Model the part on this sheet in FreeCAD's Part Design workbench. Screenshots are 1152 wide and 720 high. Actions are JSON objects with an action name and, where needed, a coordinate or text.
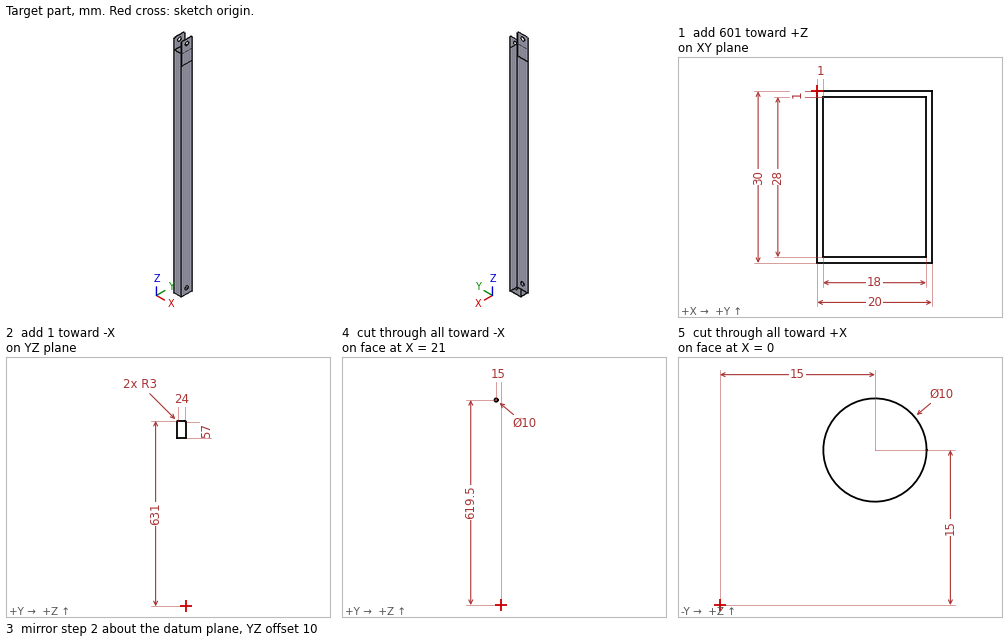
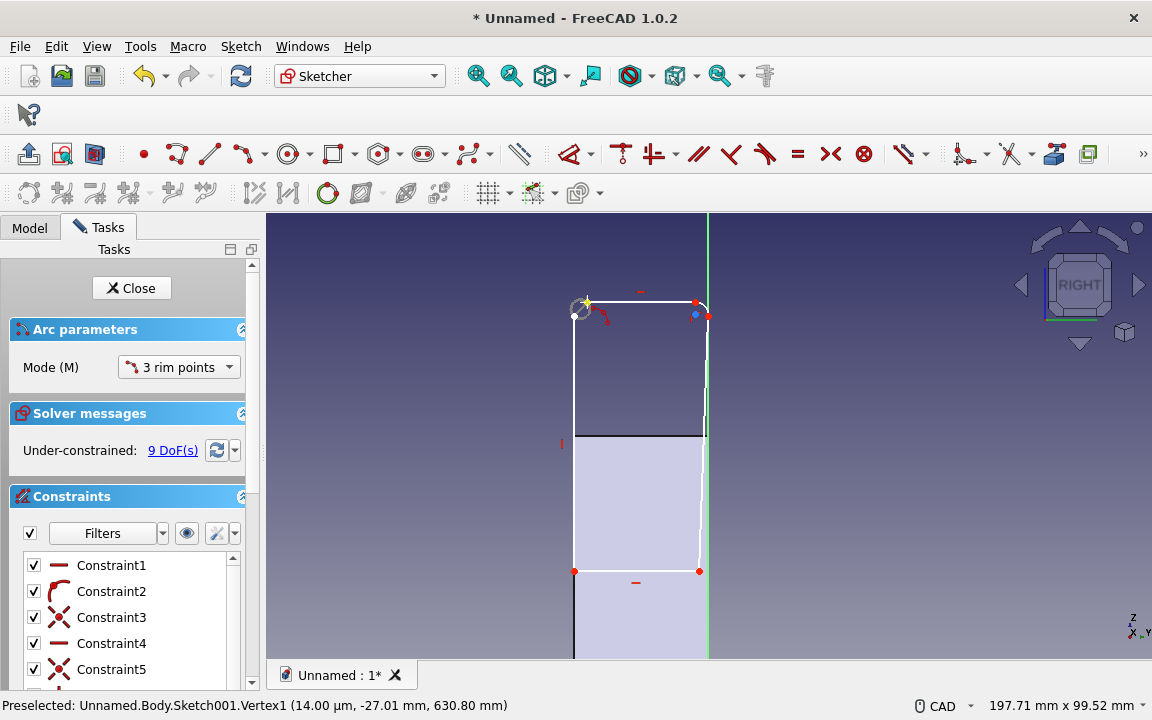
{"action": "scroll", "coordinate": [578, 305], "scroll_direction": "up", "scroll_amount": 7}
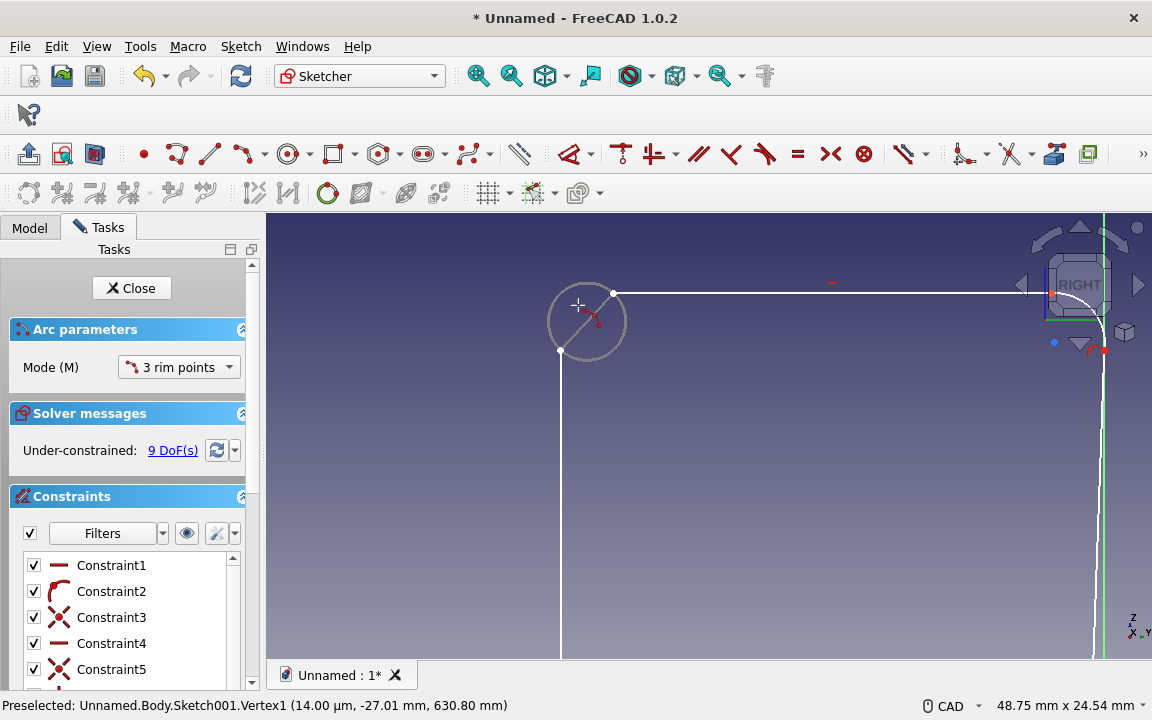
{"action": "left_click", "coordinate": [575, 306]}
{"action": "key", "text": "Escape"}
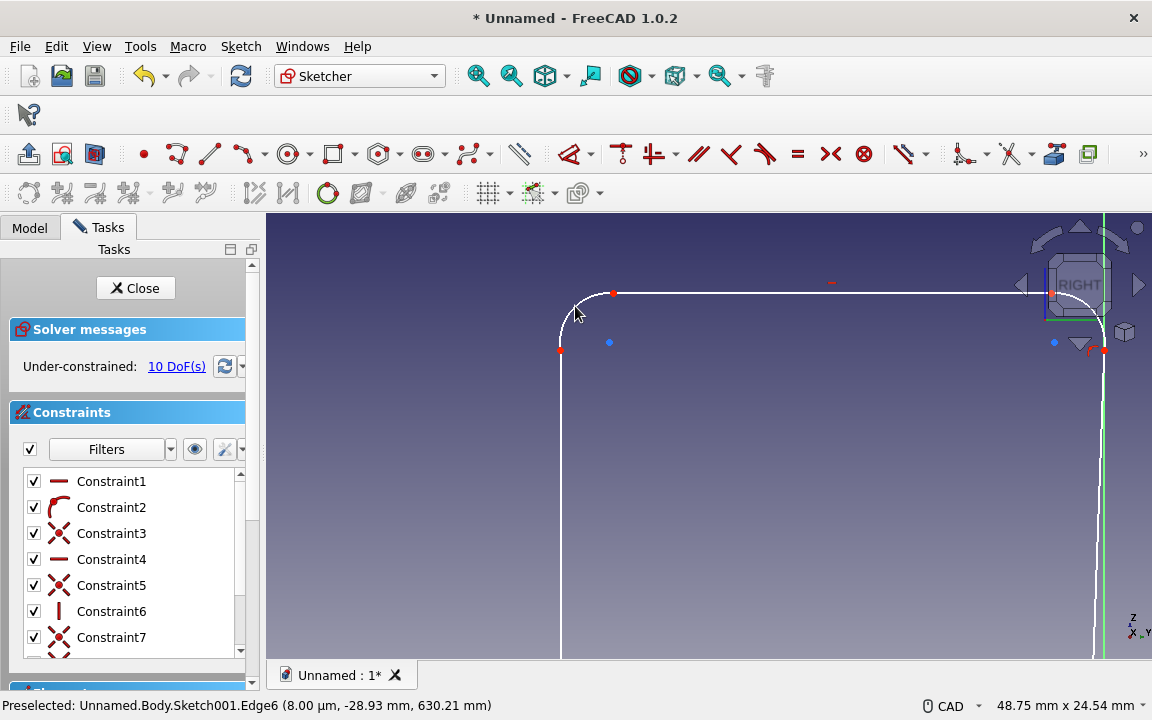
{"action": "scroll", "coordinate": [578, 305], "scroll_direction": "down", "scroll_amount": 7}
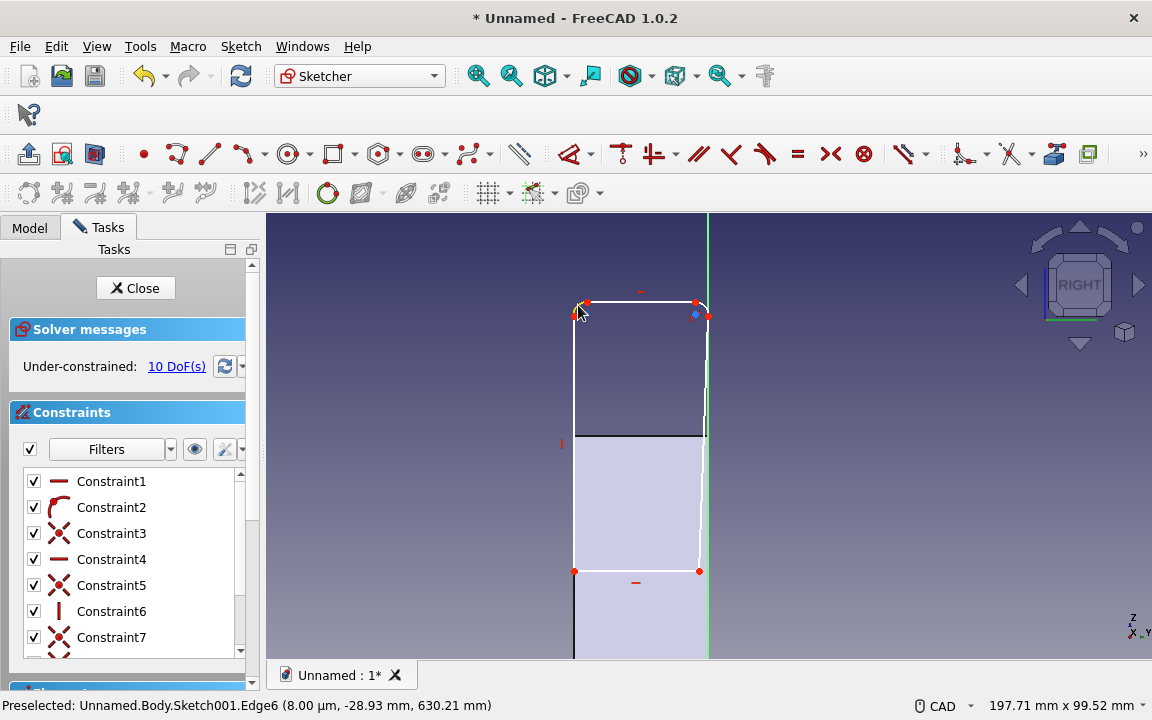
{"action": "left_click", "coordinate": [619, 302]}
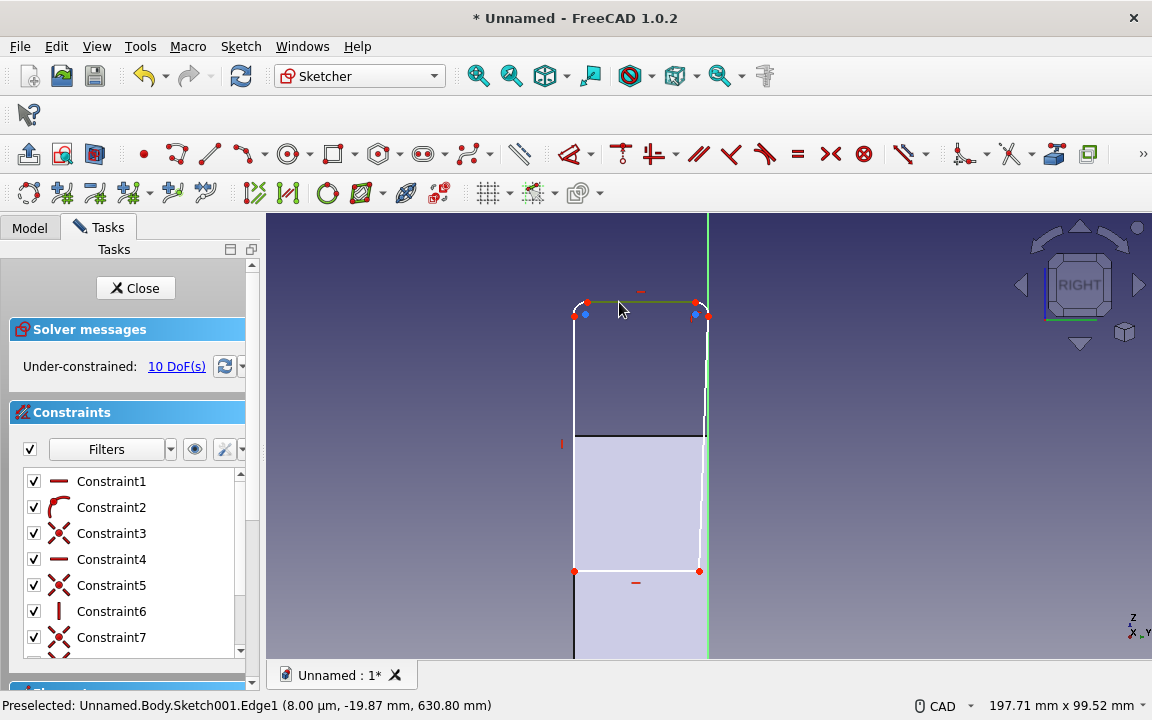
{"action": "scroll", "coordinate": [705, 306], "scroll_direction": "up", "scroll_amount": 2}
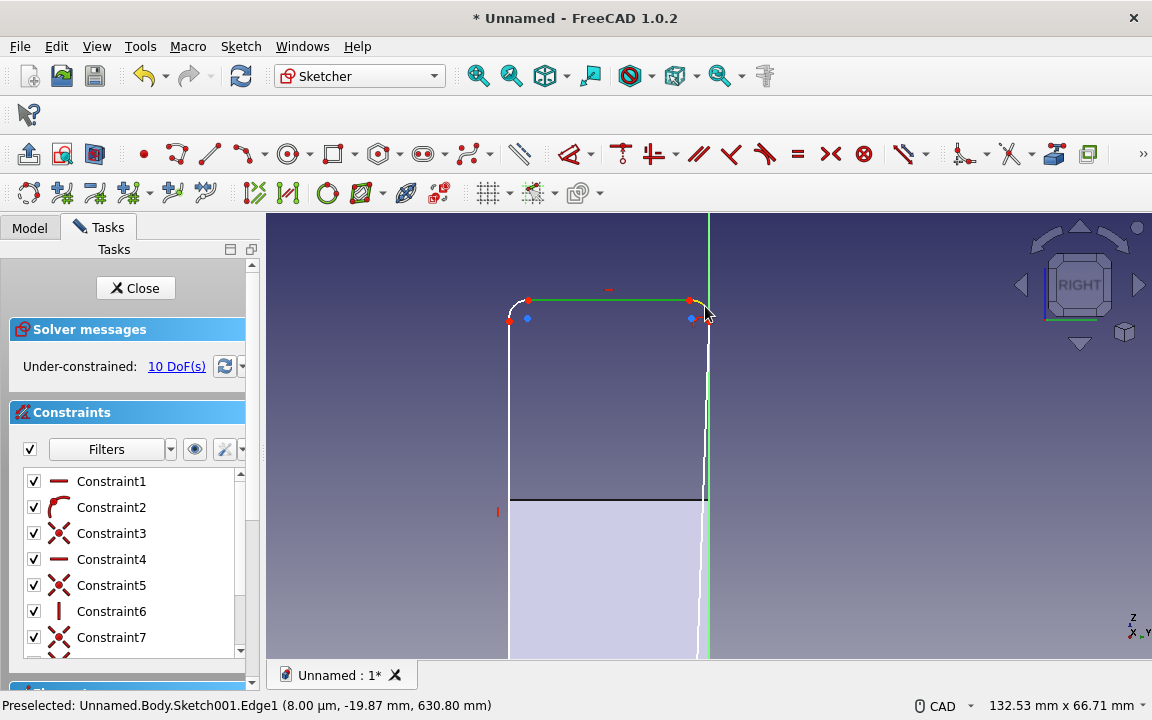
{"action": "left_click", "coordinate": [705, 306]}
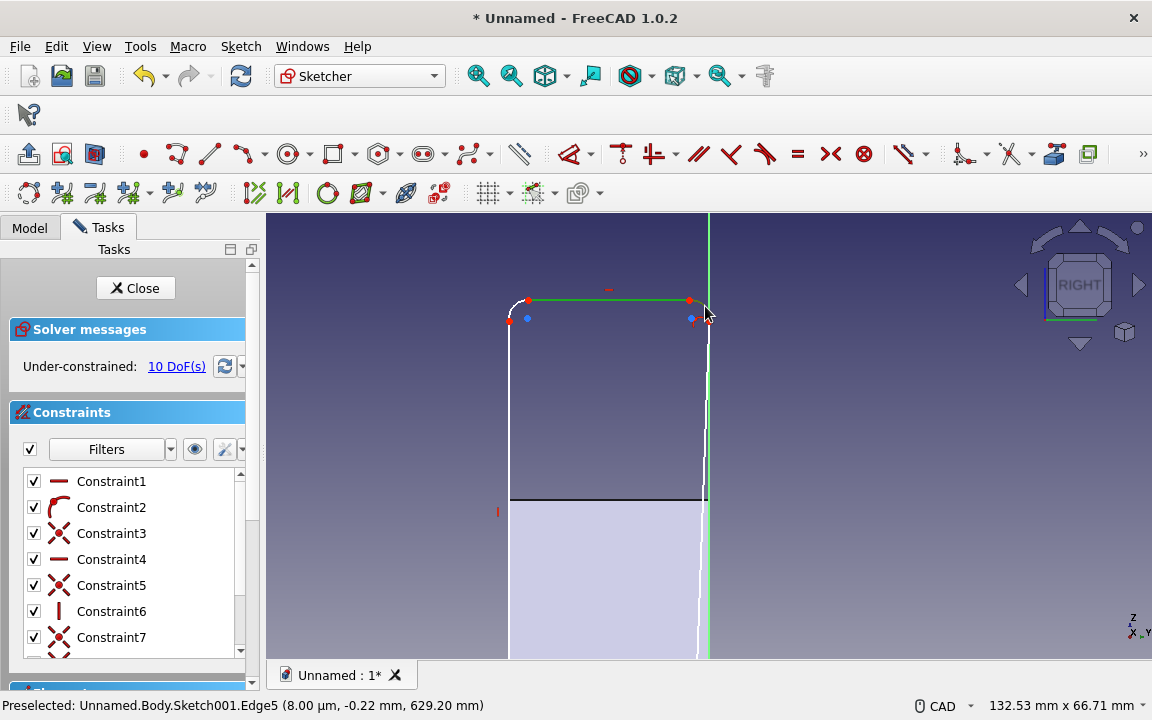
{"action": "key", "text": "t"}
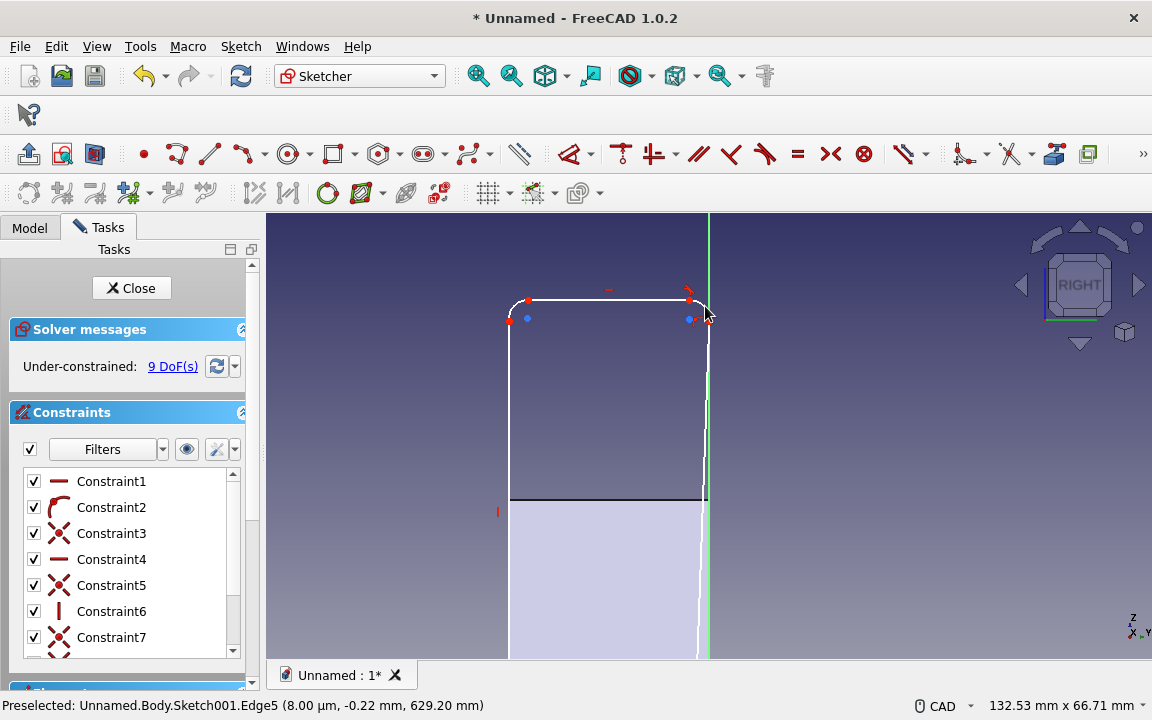
{"action": "left_click", "coordinate": [577, 300]}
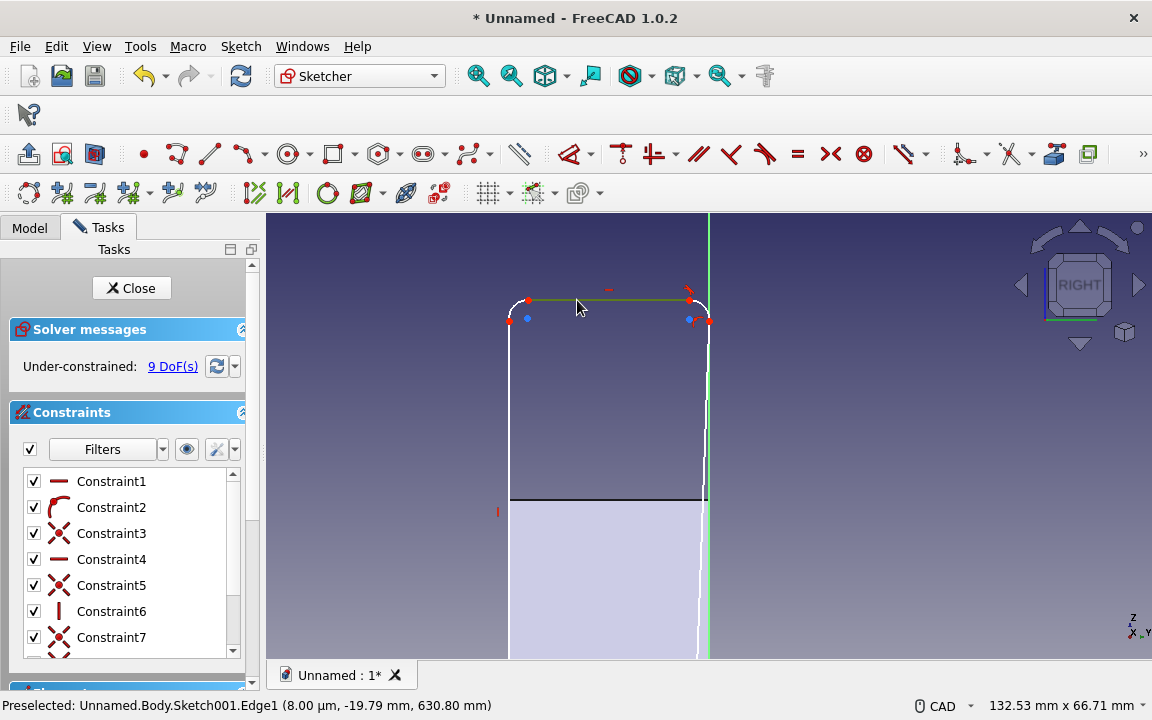
{"action": "scroll", "coordinate": [519, 302], "scroll_direction": "up", "scroll_amount": 2}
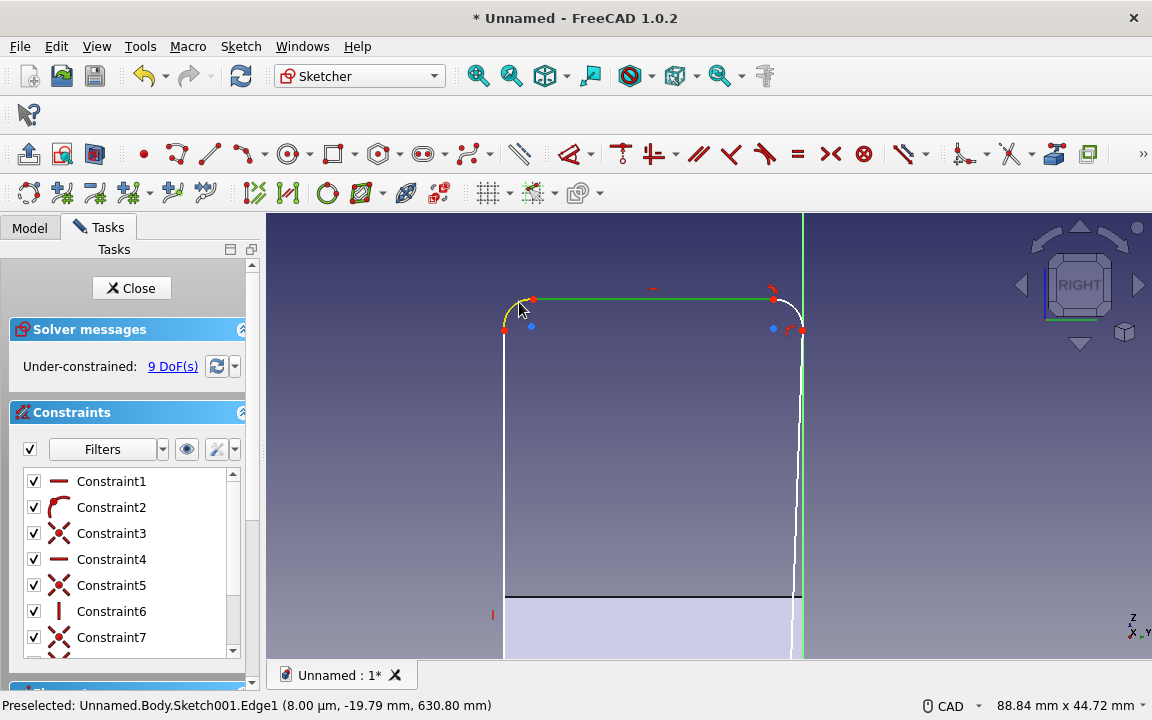
{"action": "left_click", "coordinate": [519, 302]}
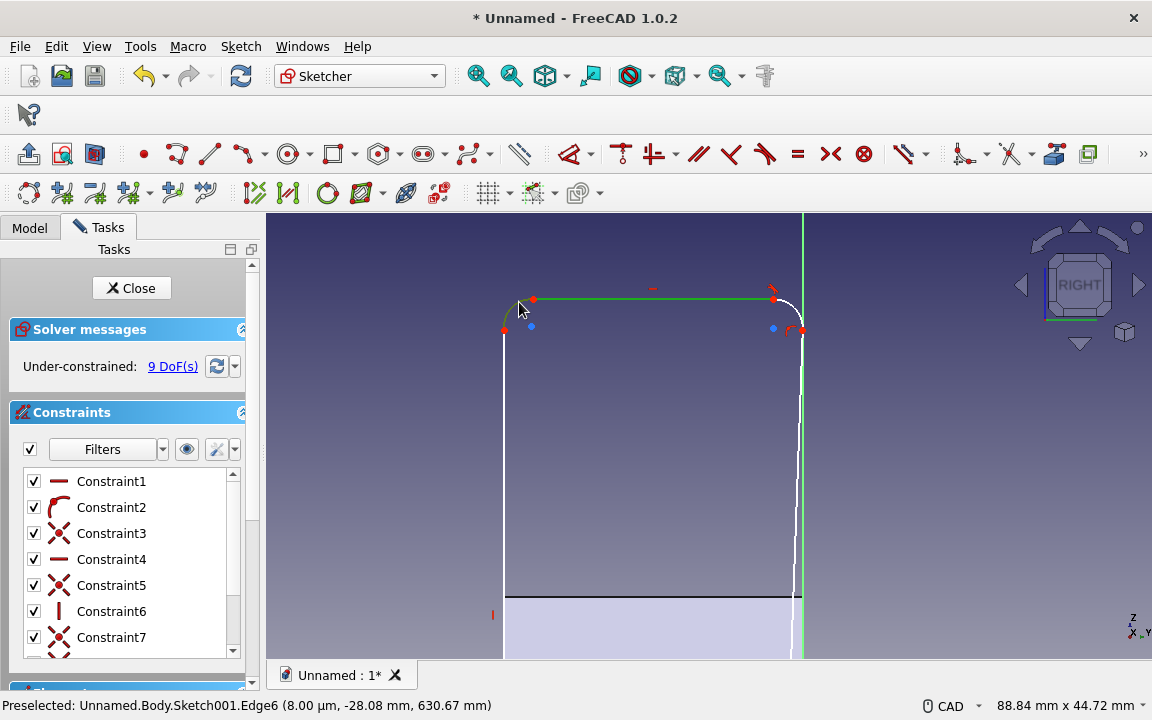
{"action": "left_click", "coordinate": [765, 154]}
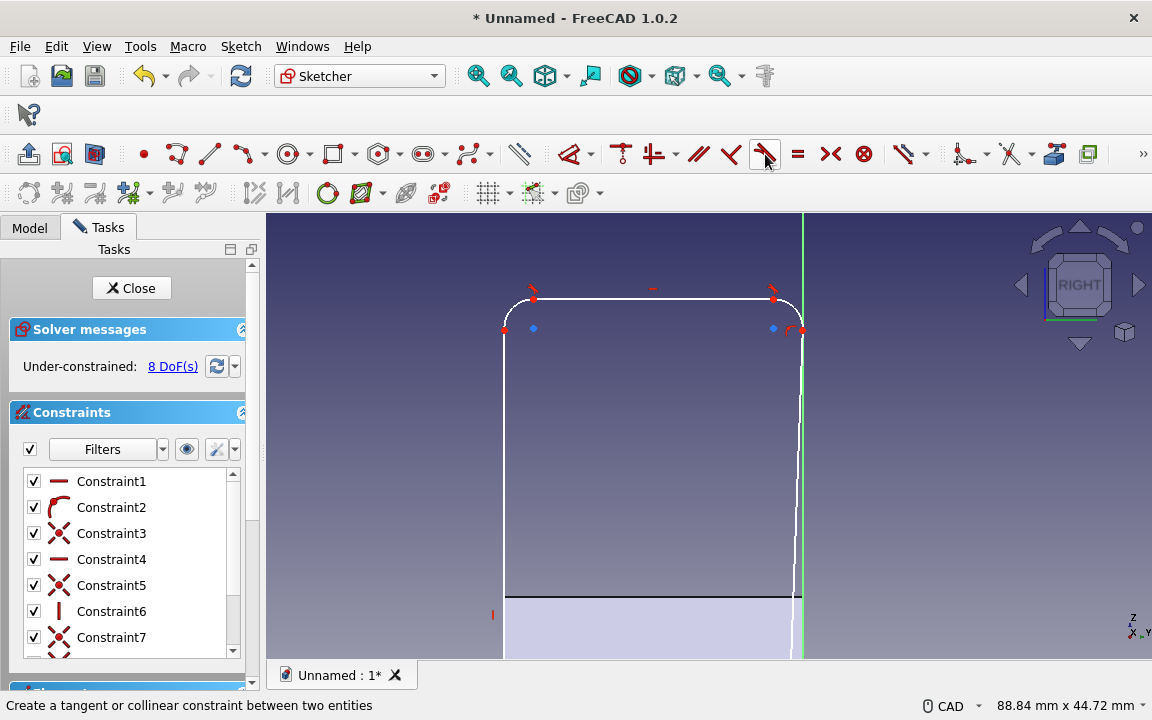
{"action": "scroll", "coordinate": [793, 614], "scroll_direction": "up", "scroll_amount": 2}